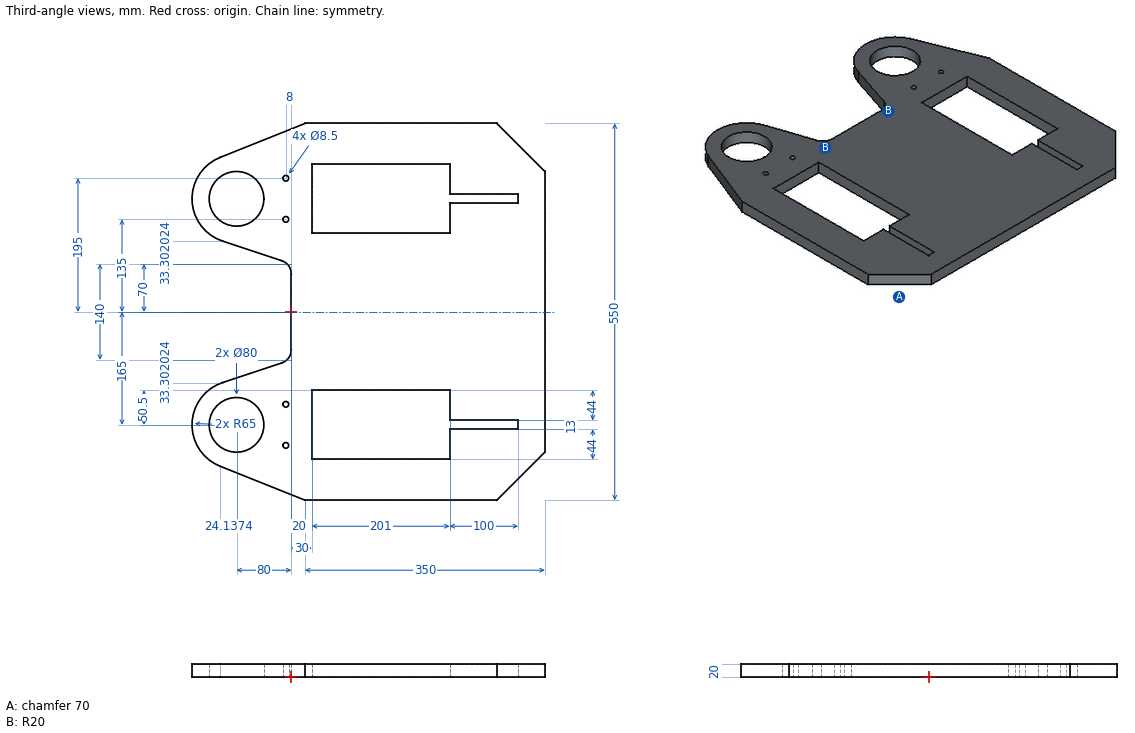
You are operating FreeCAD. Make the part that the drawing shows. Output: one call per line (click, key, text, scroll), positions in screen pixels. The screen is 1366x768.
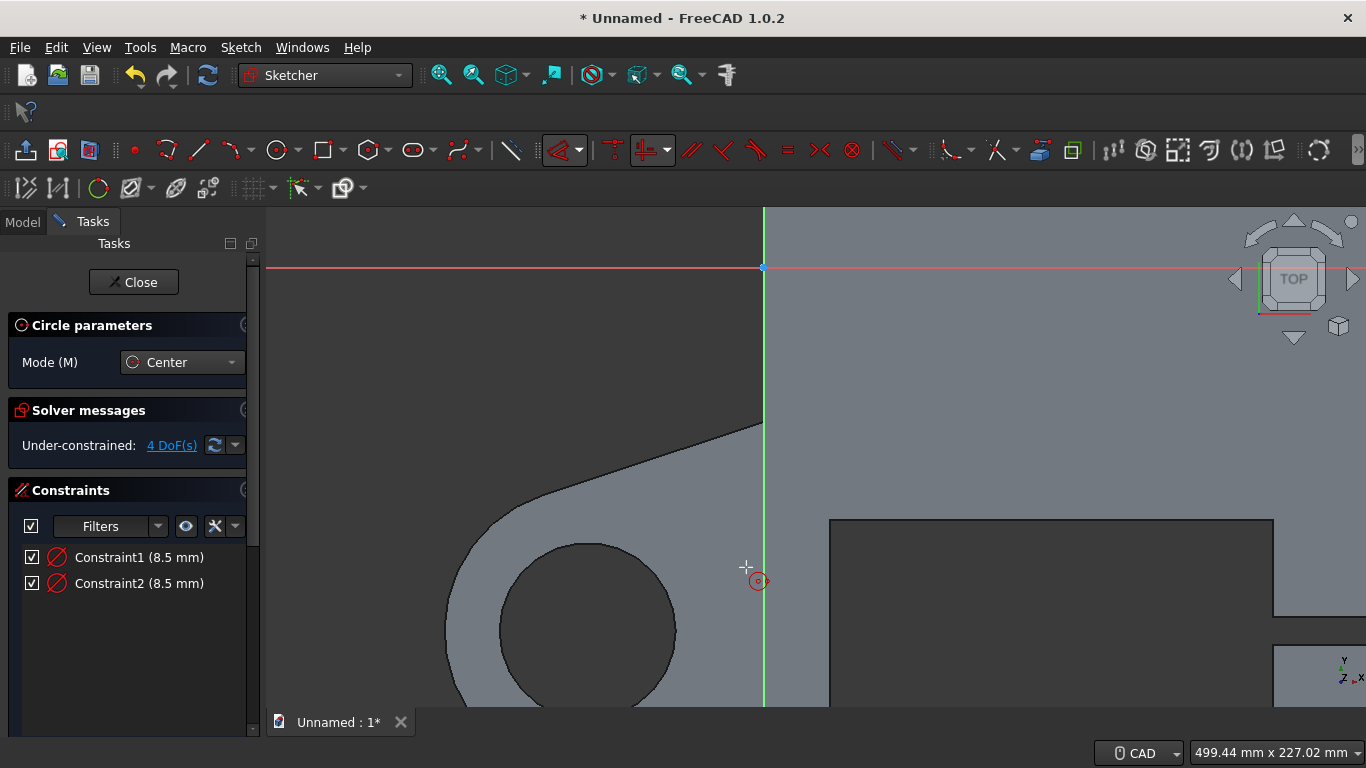
click(746, 565)
move(740, 558)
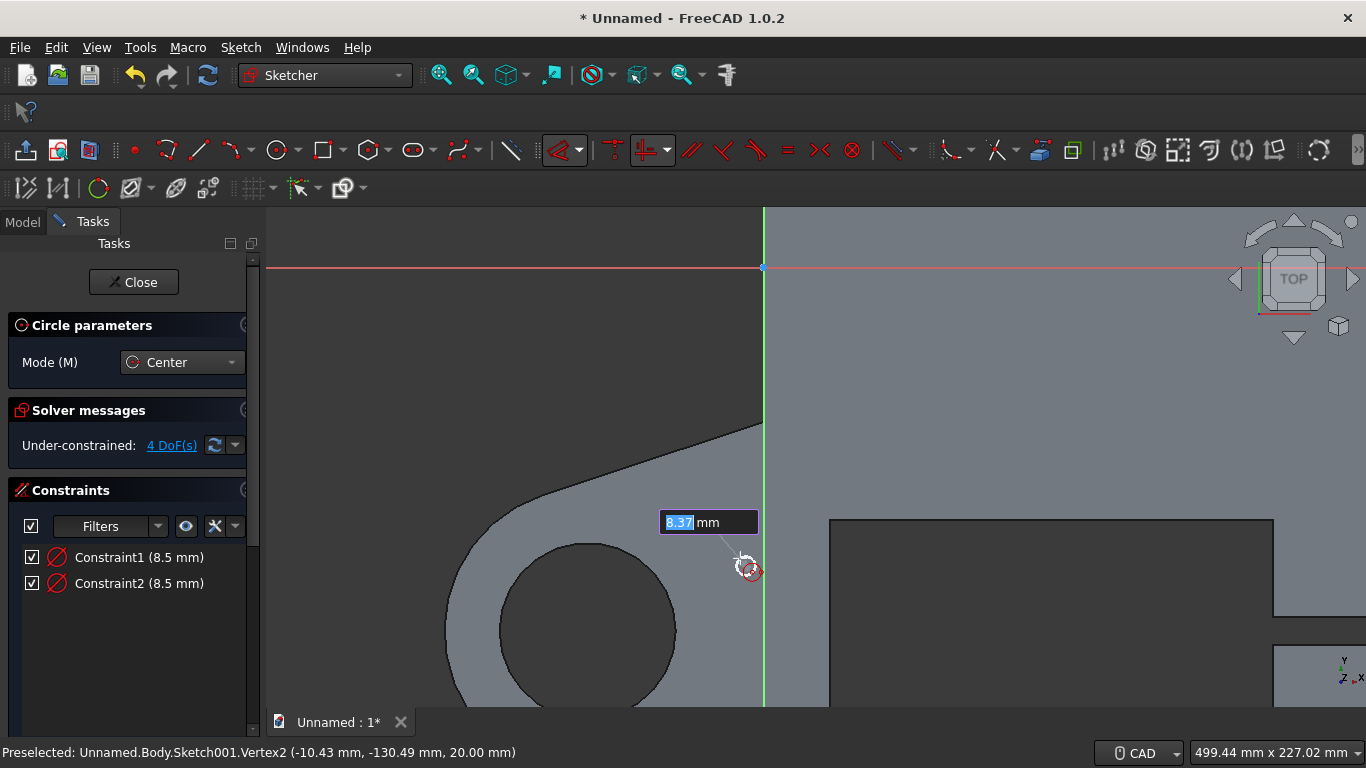
text(8.5)
key(Return)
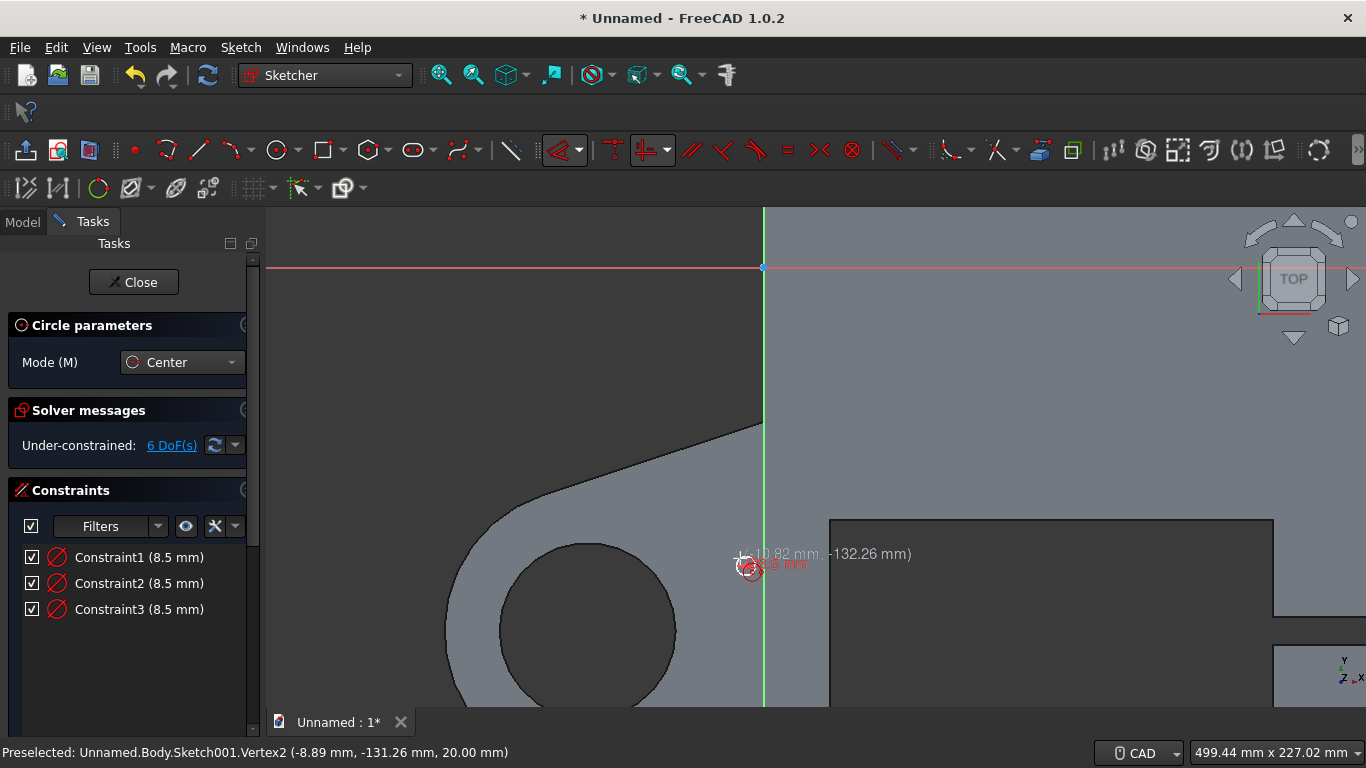
scroll(746, 567, down, 5)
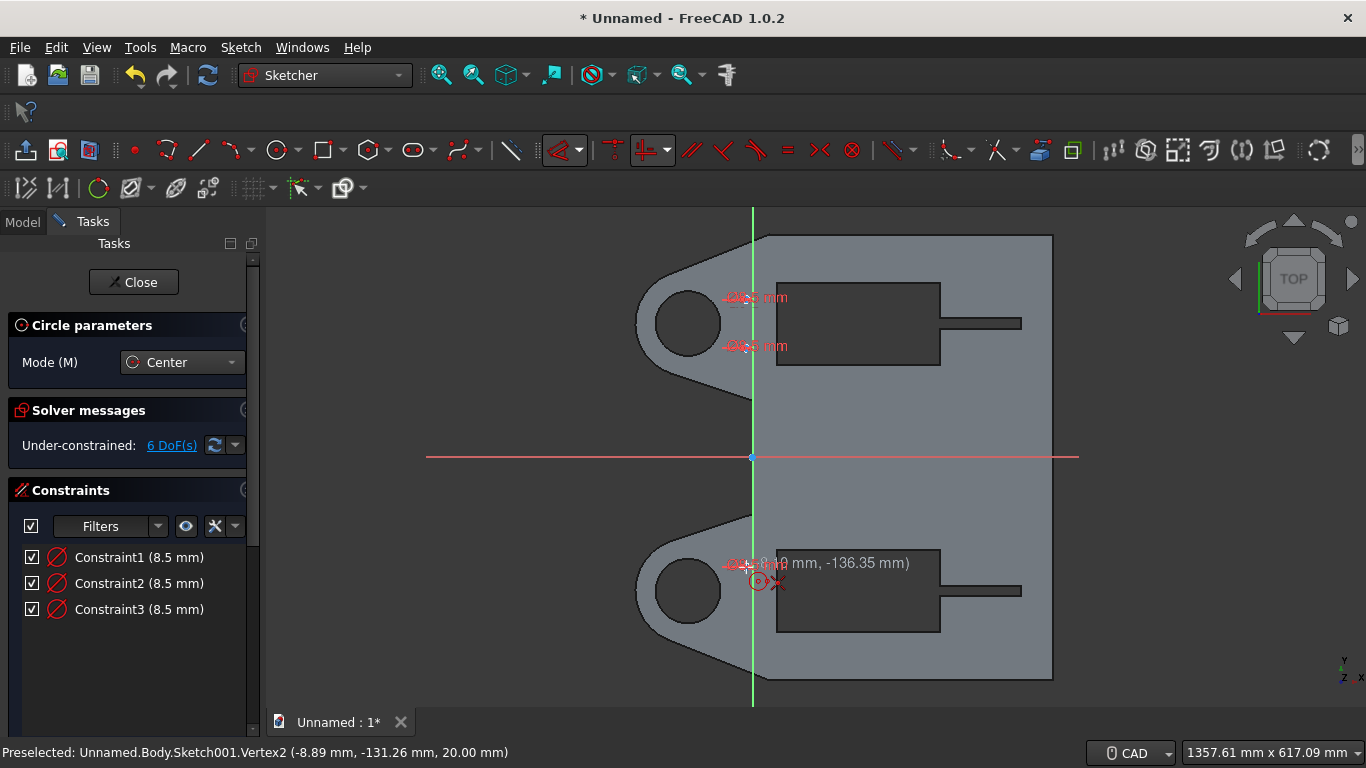
scroll(746, 615, up, 10)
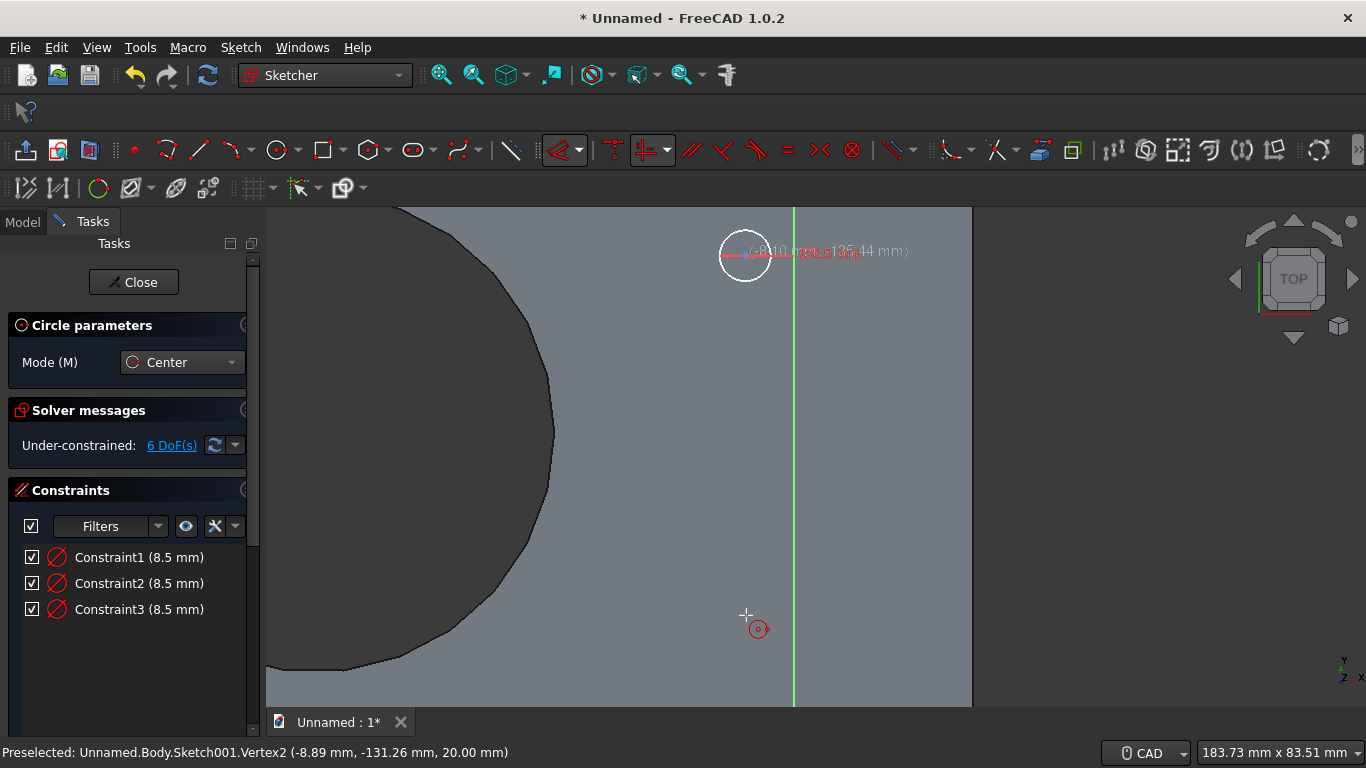
scroll(746, 615, down, 10)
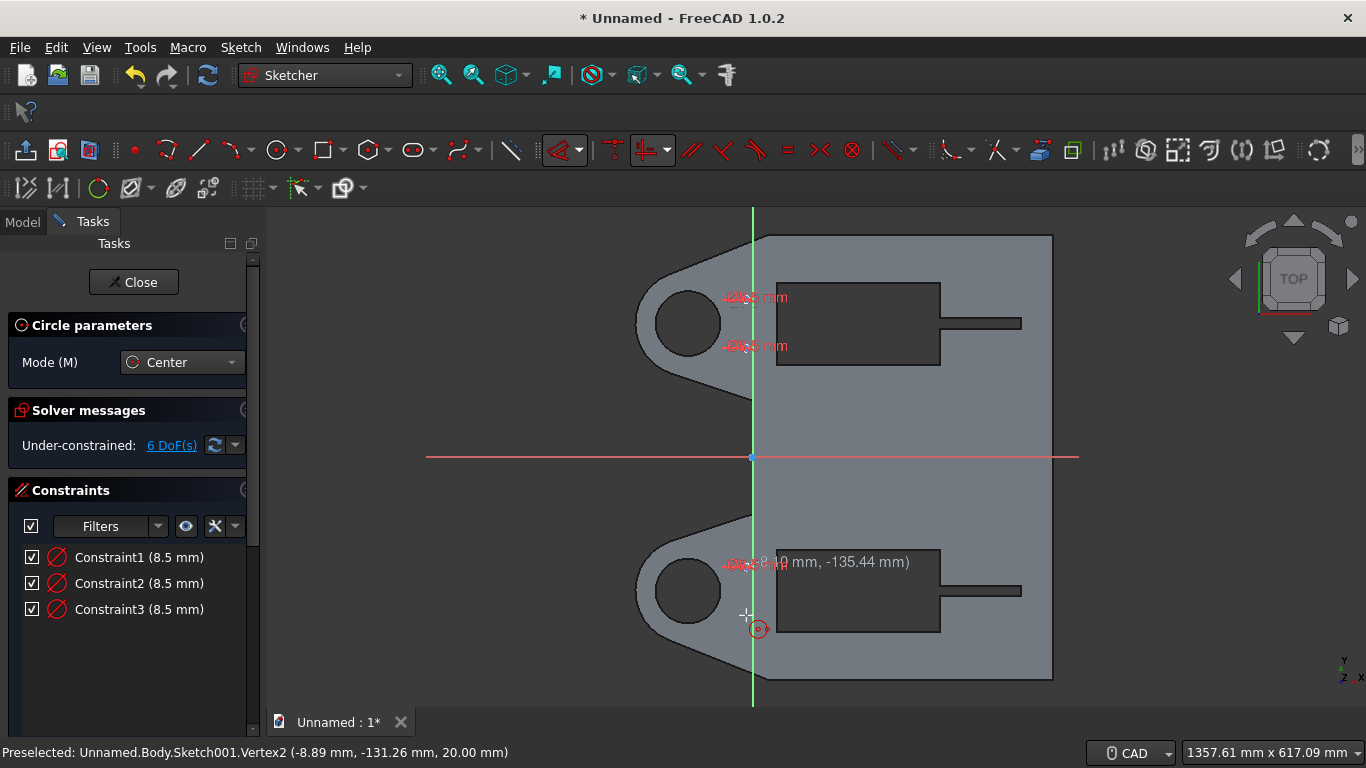
scroll(746, 615, up, 5)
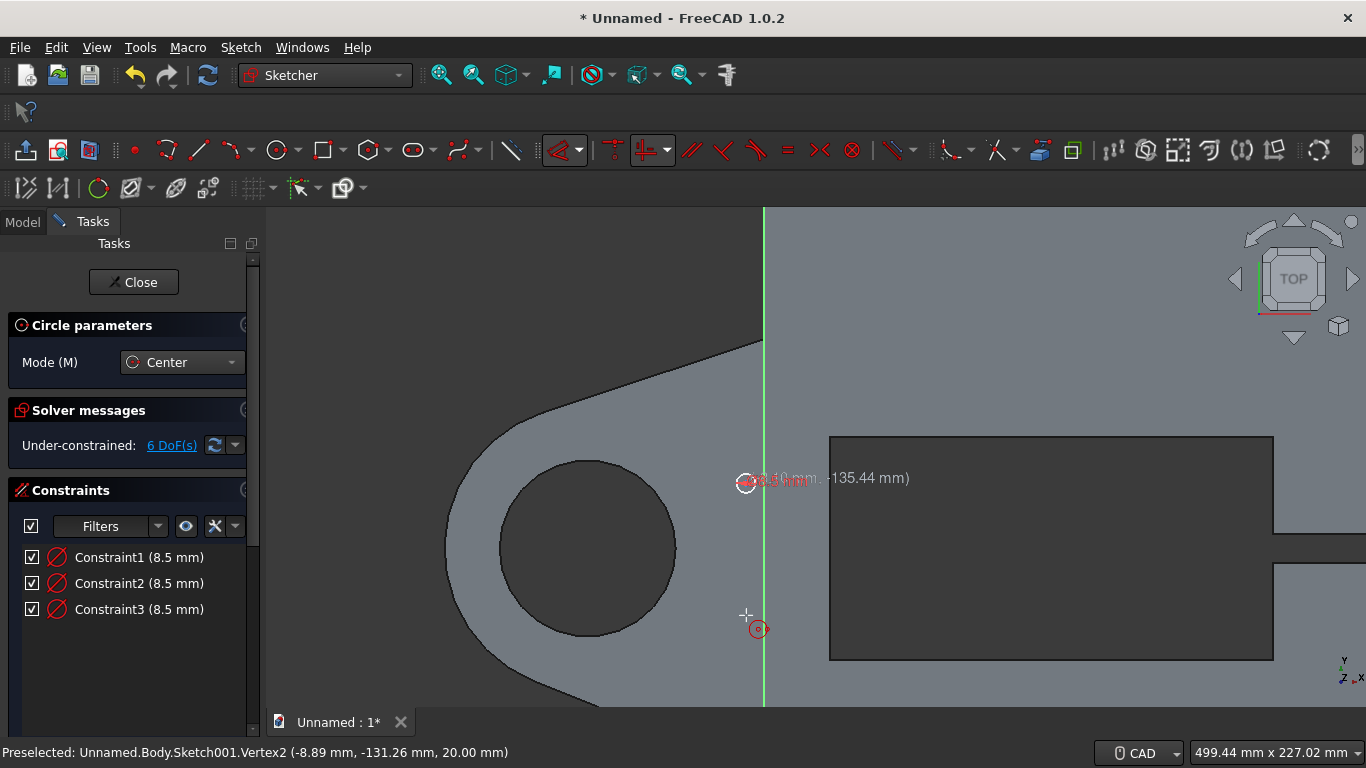
click(746, 615)
move(740, 608)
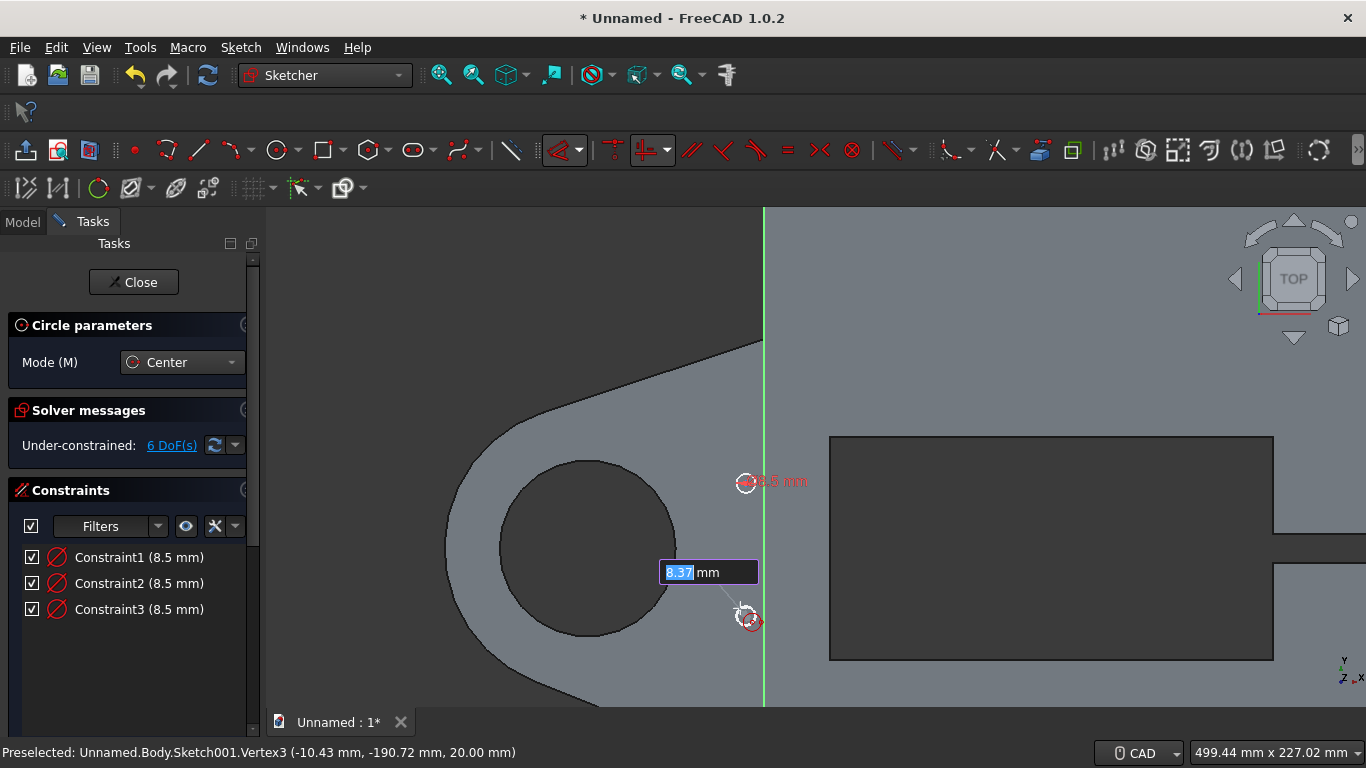
text(8.5)
key(Return)
key(Escape)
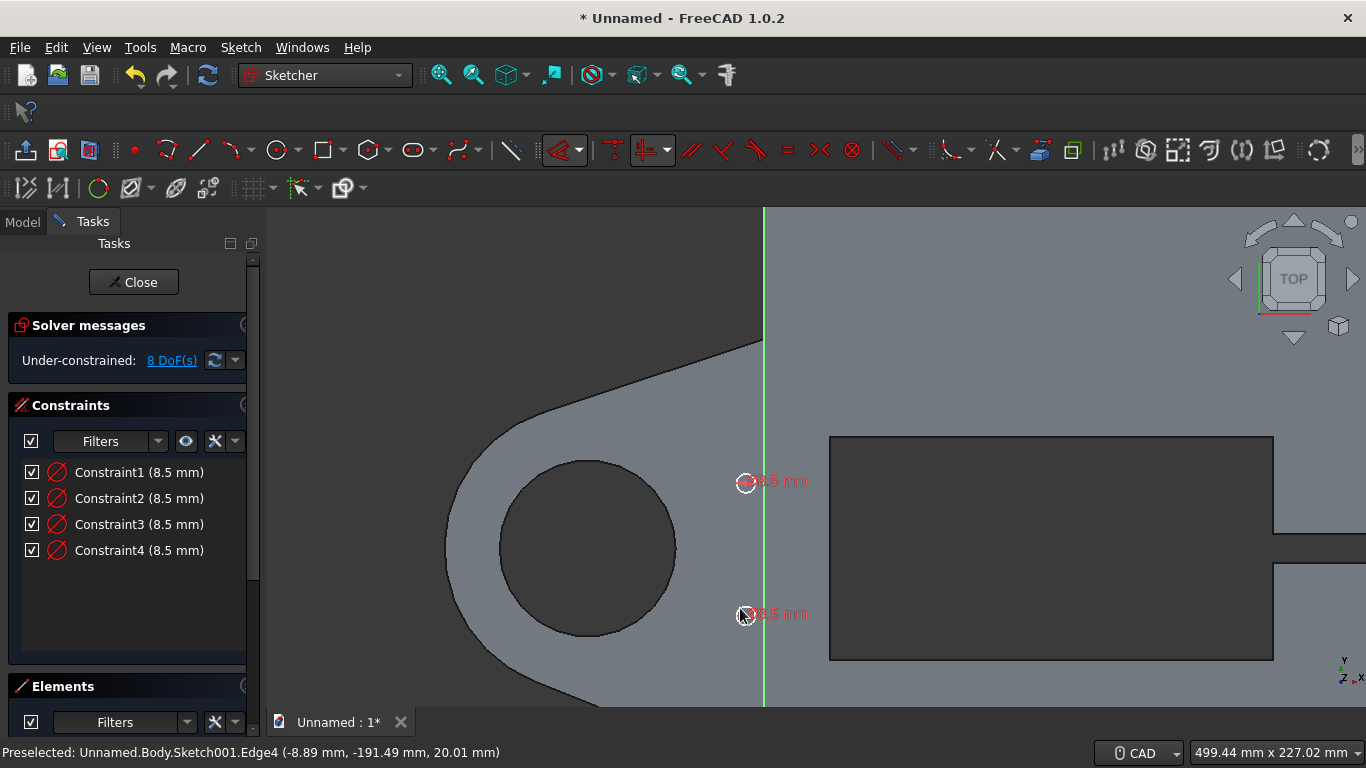
scroll(746, 615, down, 5)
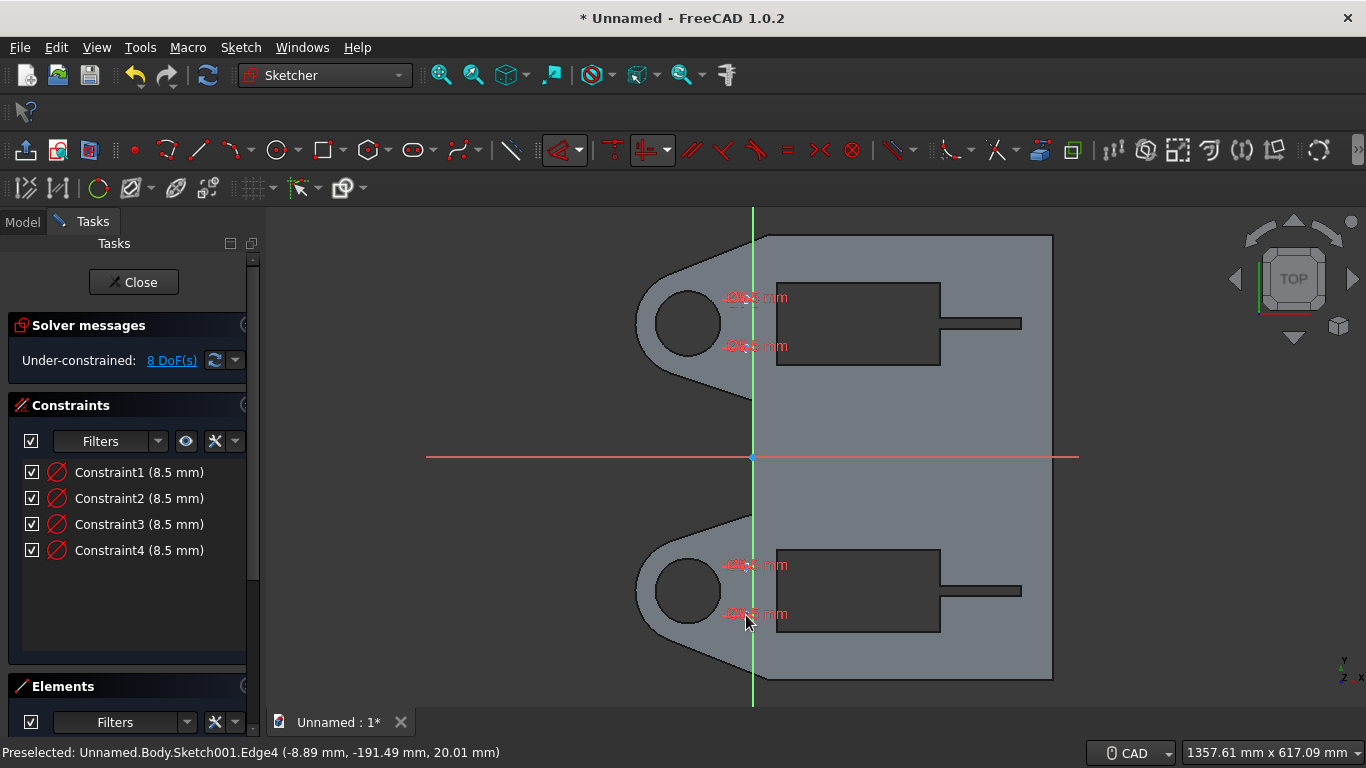
click(746, 348)